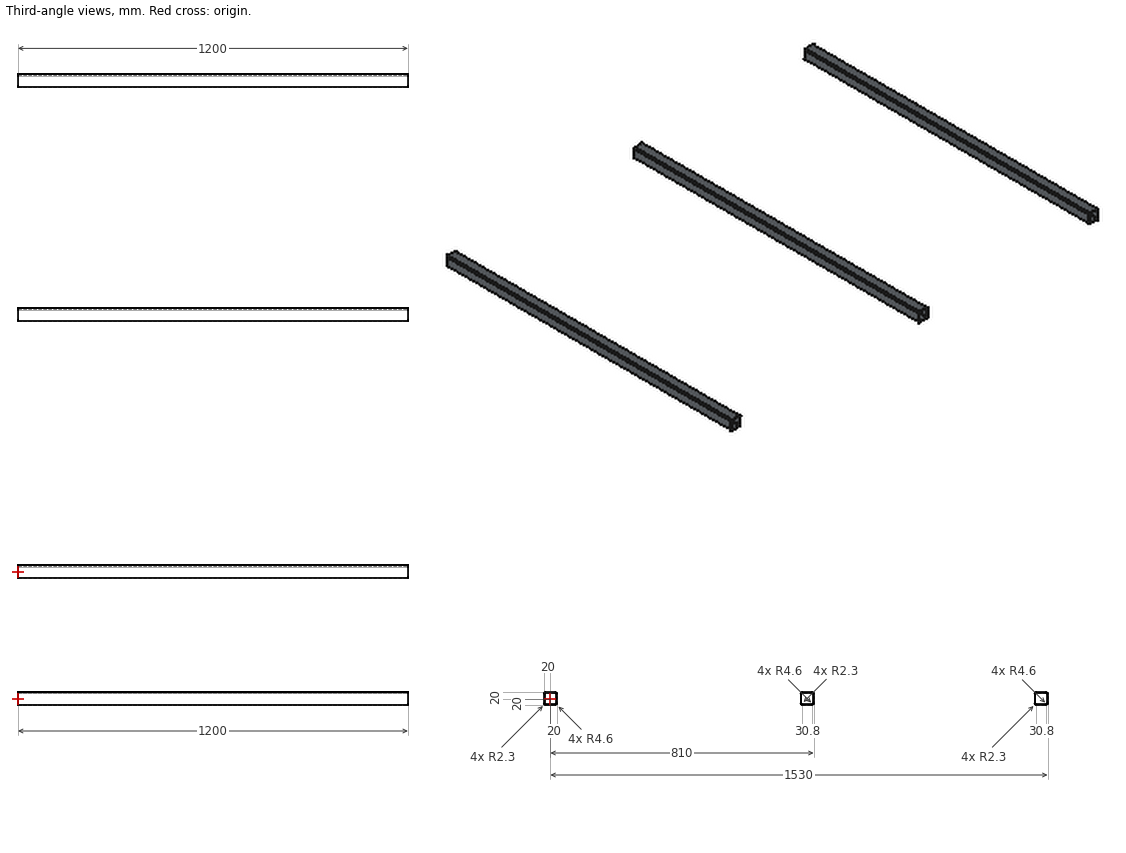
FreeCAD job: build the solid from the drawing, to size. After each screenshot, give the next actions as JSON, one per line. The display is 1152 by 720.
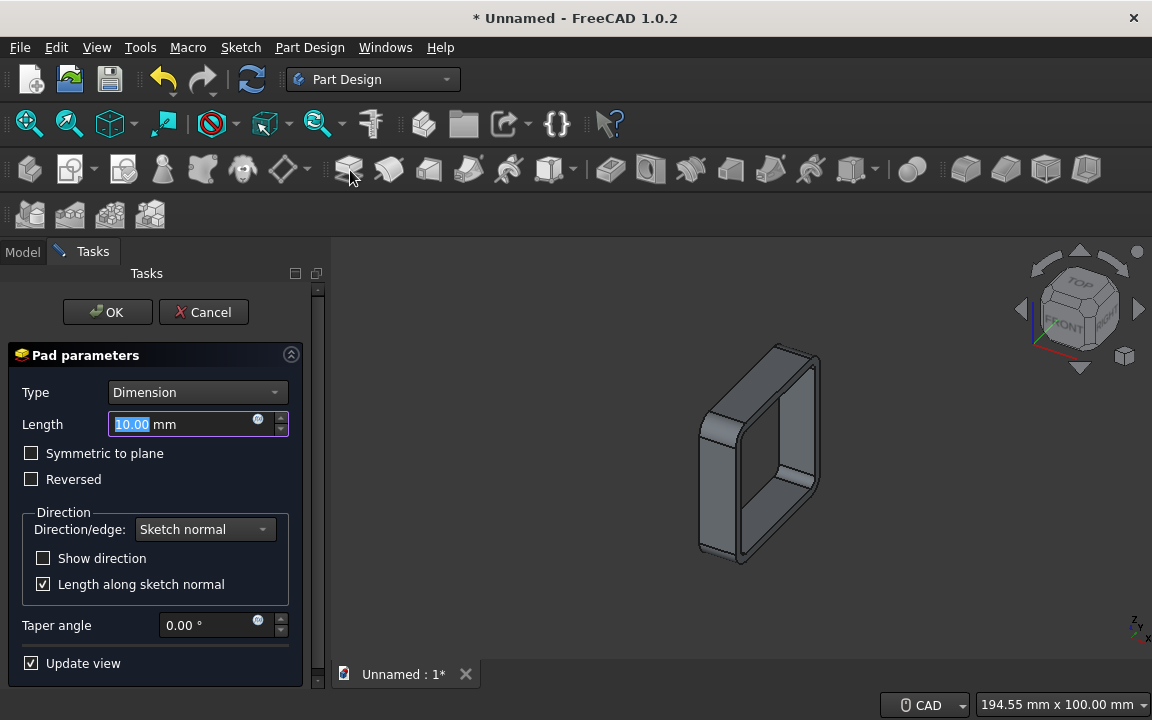
{"action": "type", "text": "1200"}
{"action": "key", "text": "Tab"}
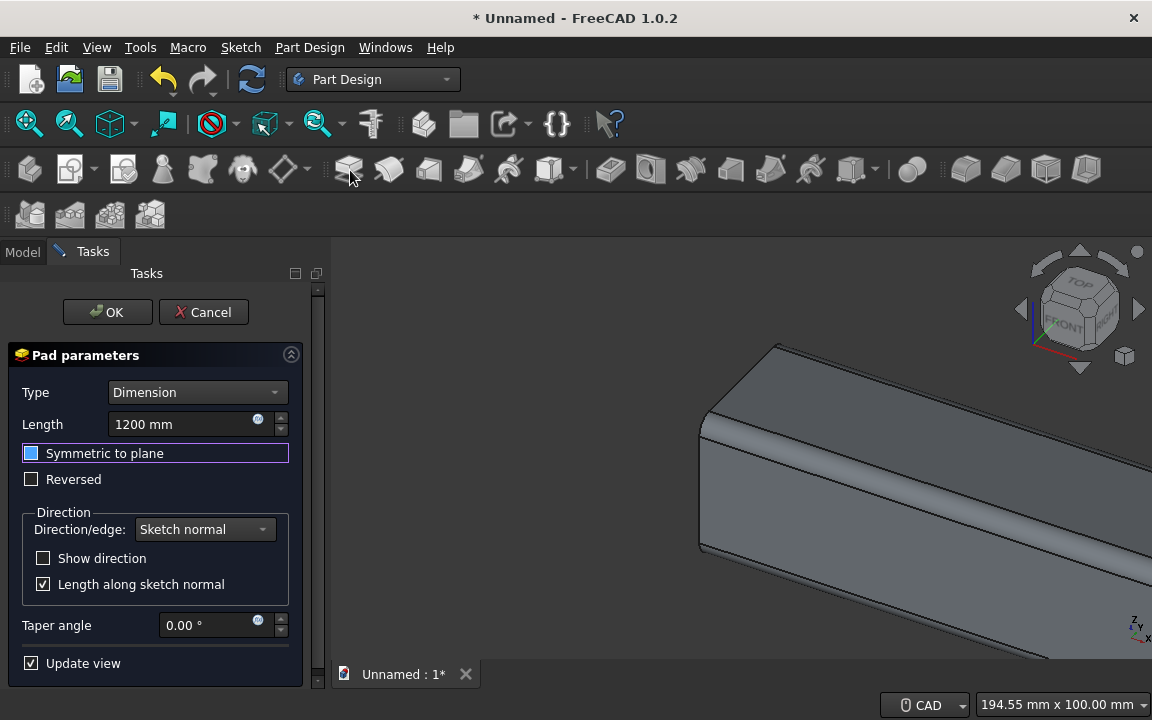
{"action": "left_click", "coordinate": [108, 312]}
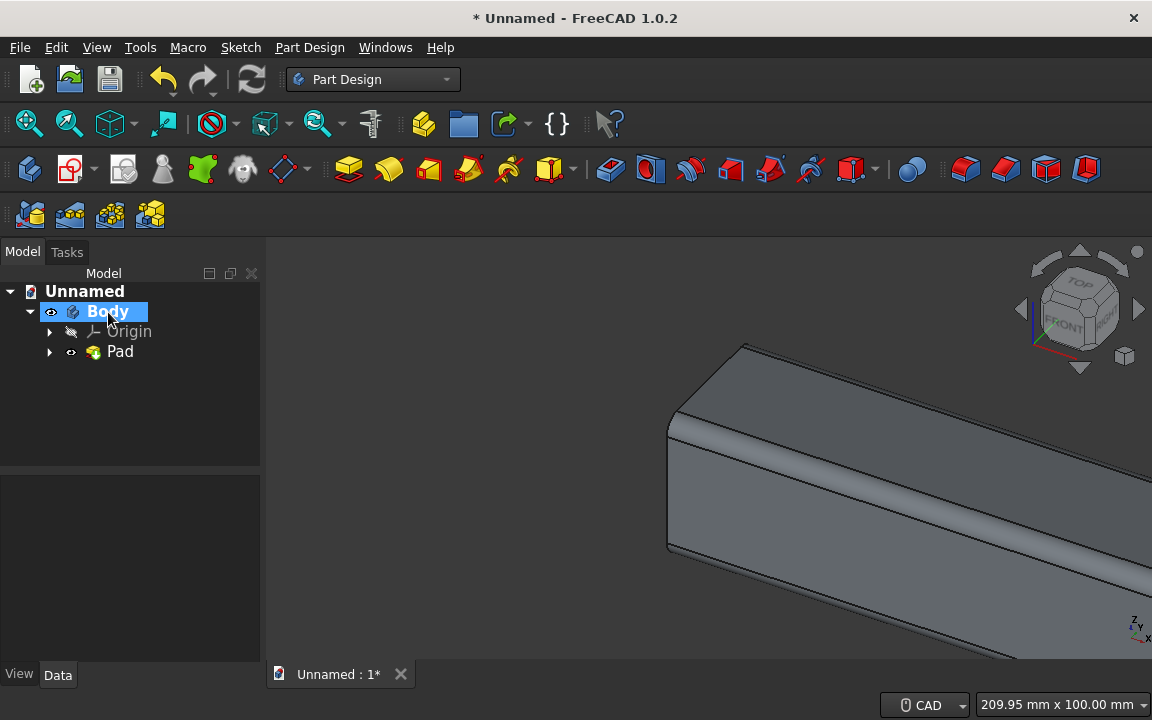
{"action": "key", "text": "v f"}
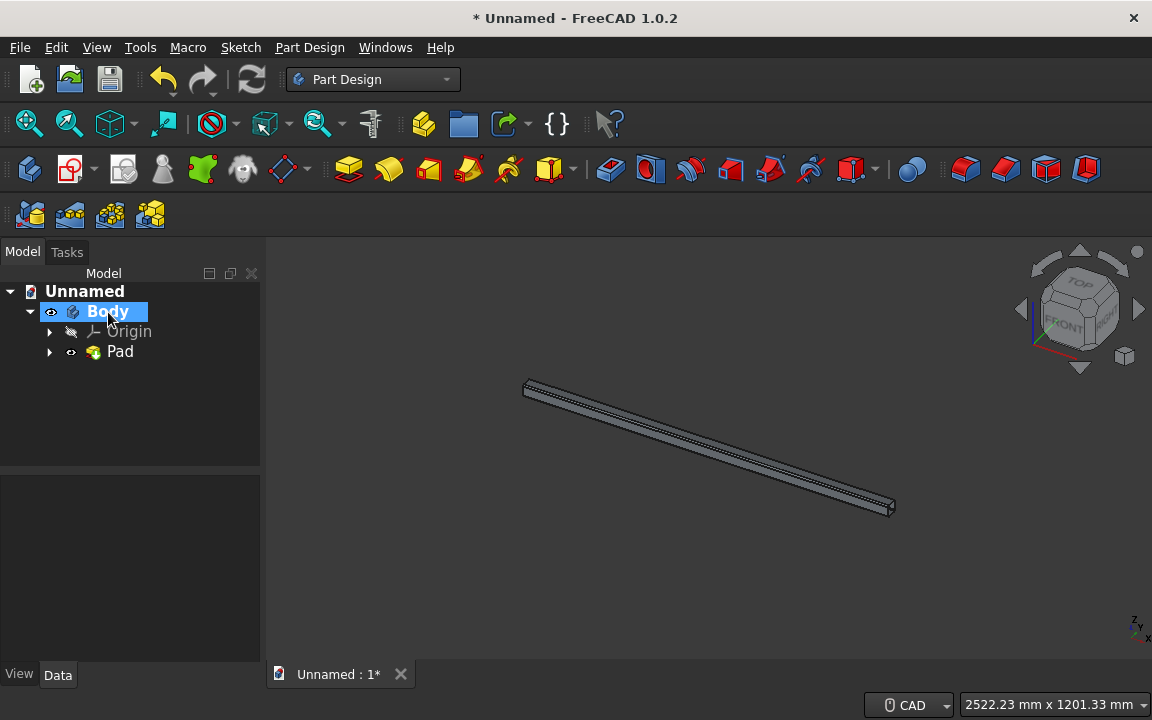
{"action": "left_click", "coordinate": [30, 170]}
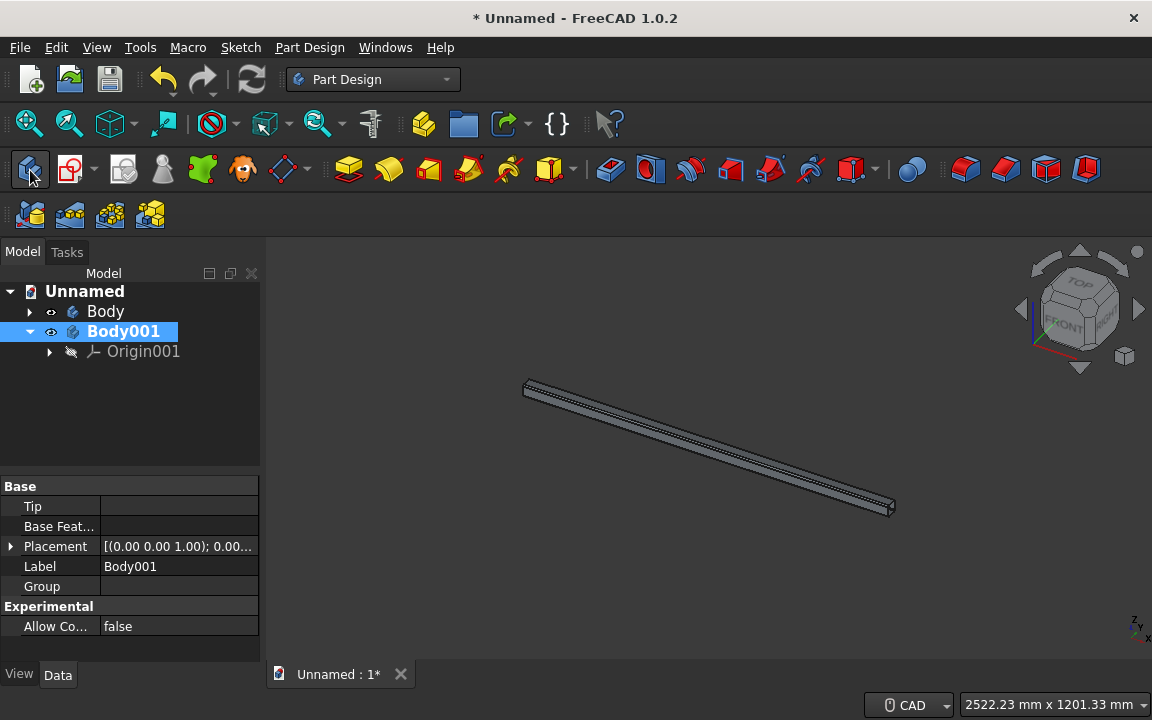
{"action": "left_click", "coordinate": [306, 619]}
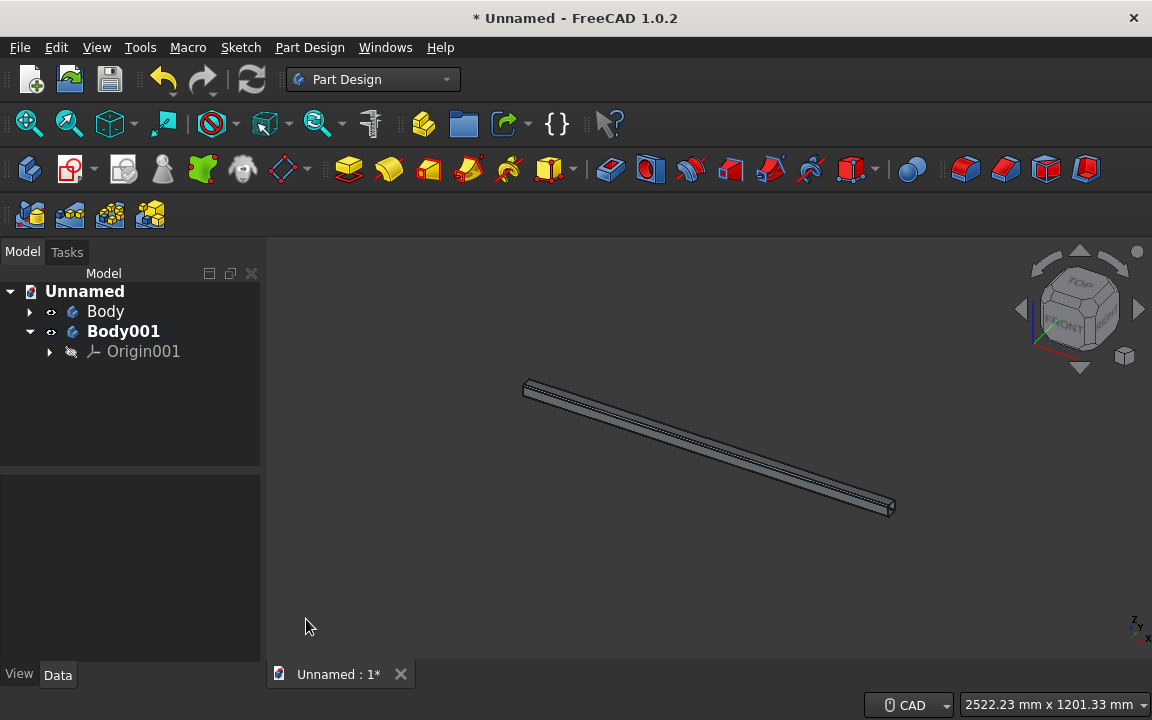
{"action": "left_click", "coordinate": [70, 170]}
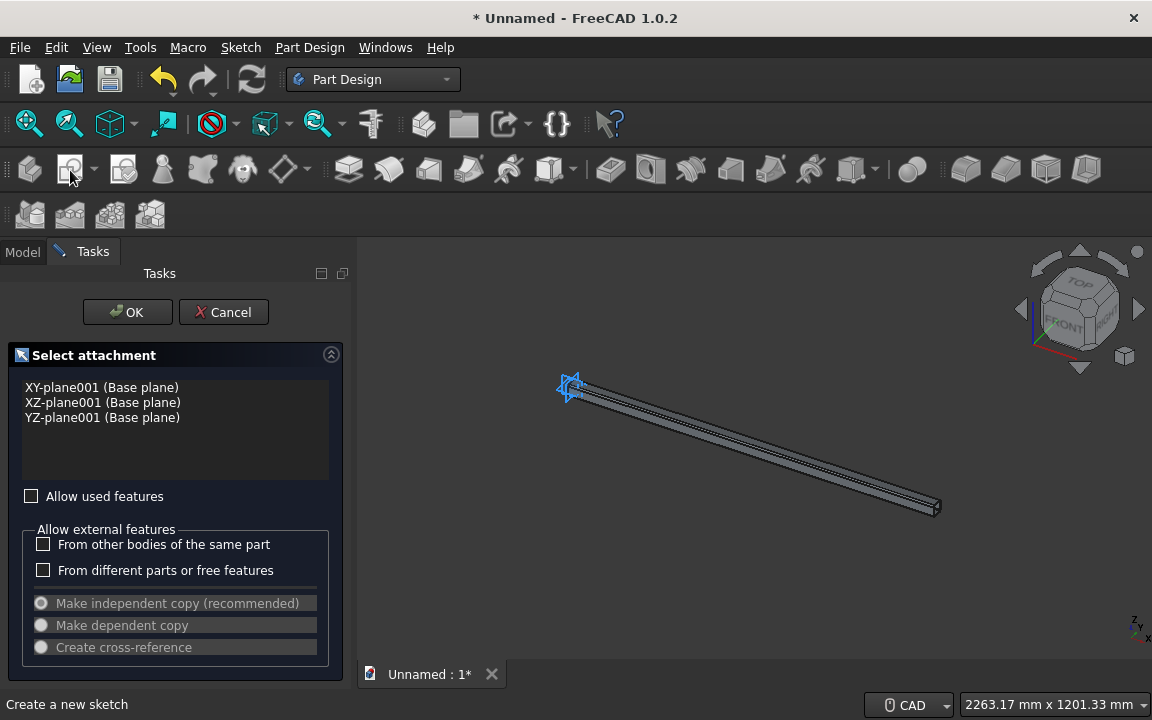
{"action": "left_click", "coordinate": [82, 418]}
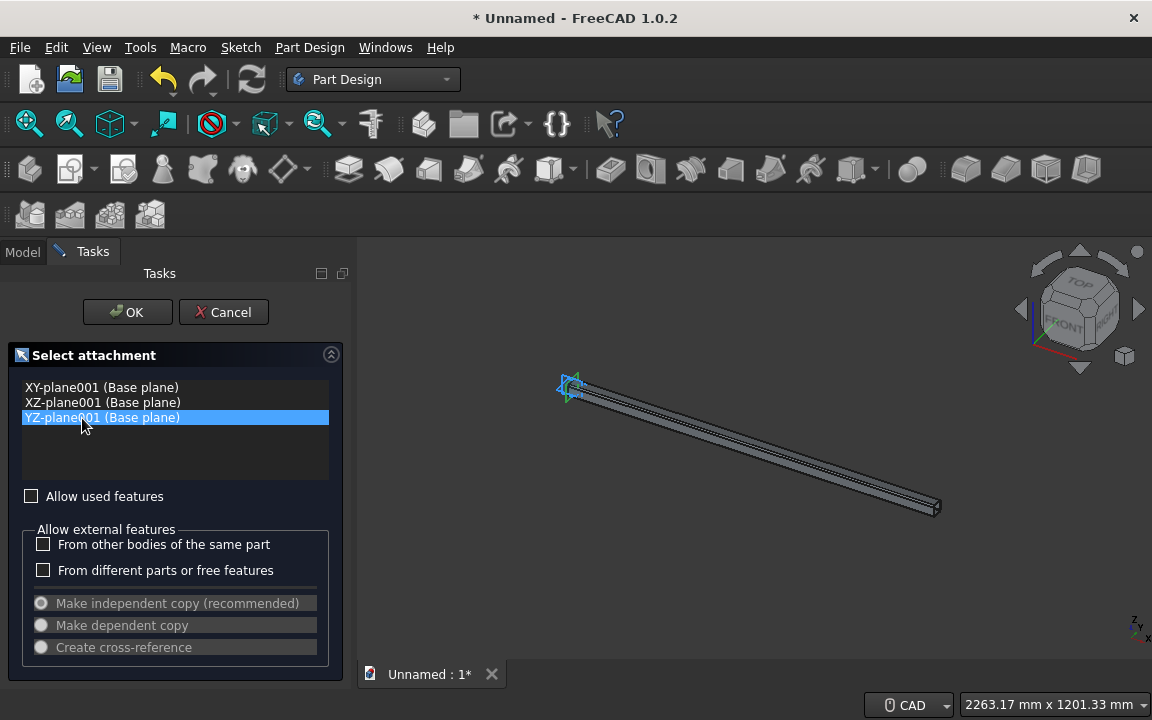
{"action": "left_click", "coordinate": [128, 312]}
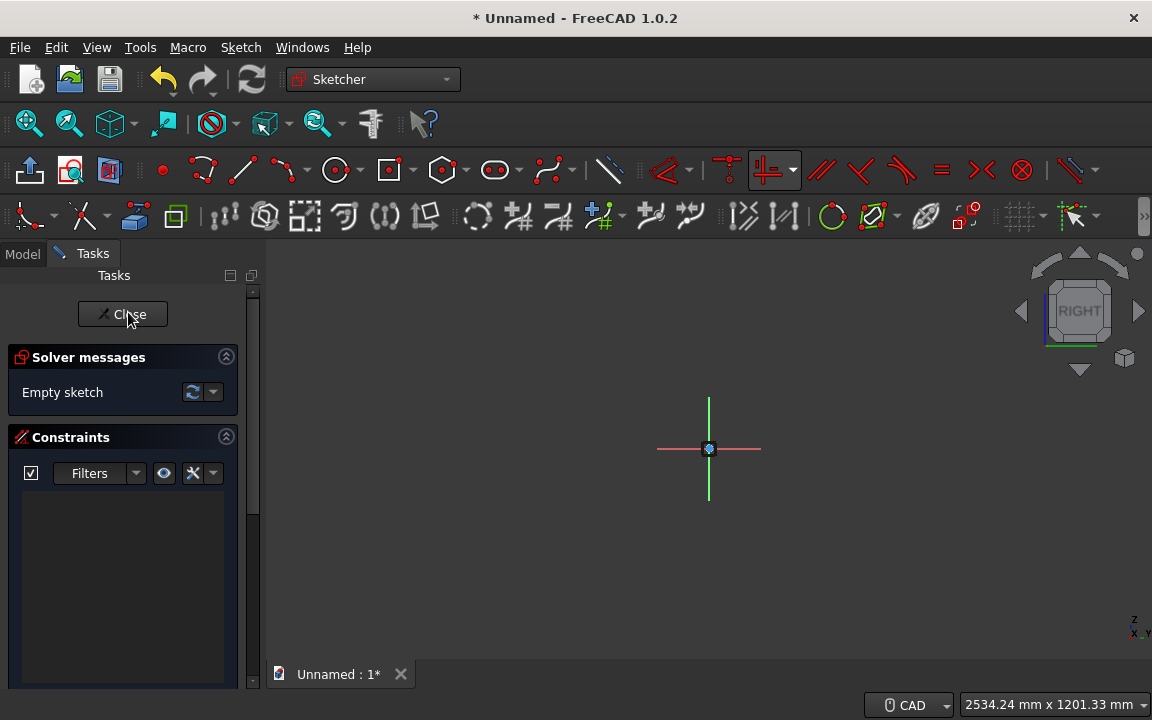
{"action": "scroll", "coordinate": [640, 449], "scroll_direction": "down", "scroll_amount": 5}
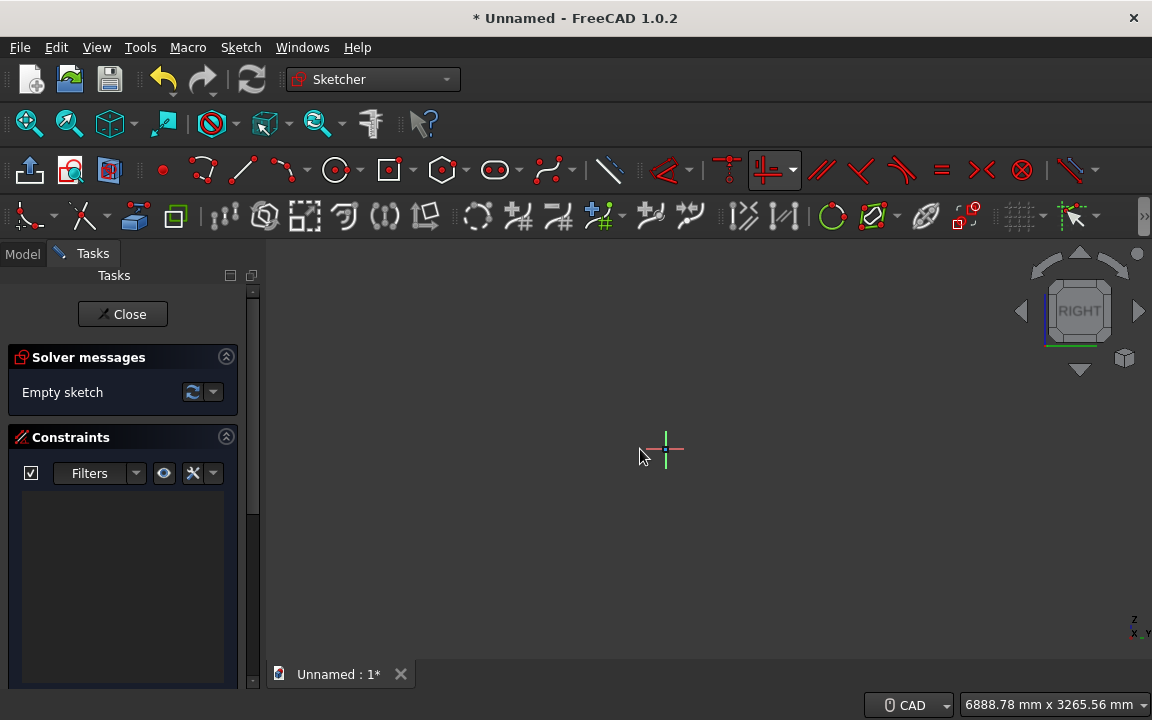
{"action": "scroll", "coordinate": [871, 449], "scroll_direction": "up", "scroll_amount": 15}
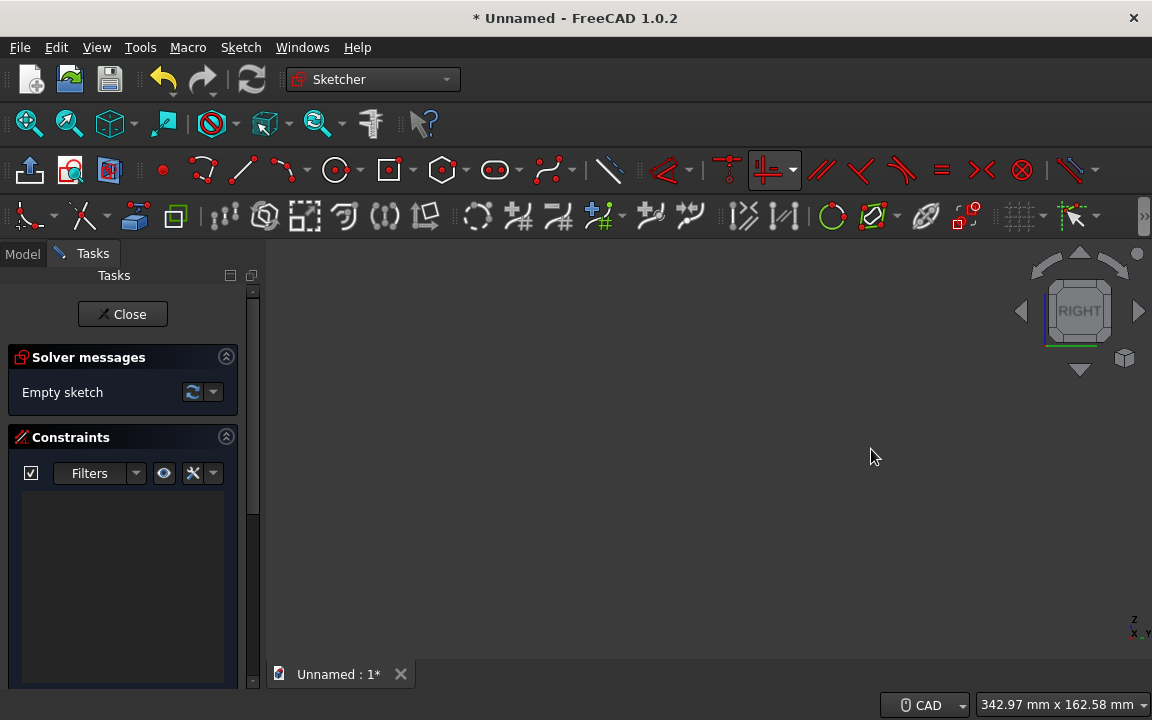
{"action": "scroll", "coordinate": [631, 444], "scroll_direction": "up", "scroll_amount": 5}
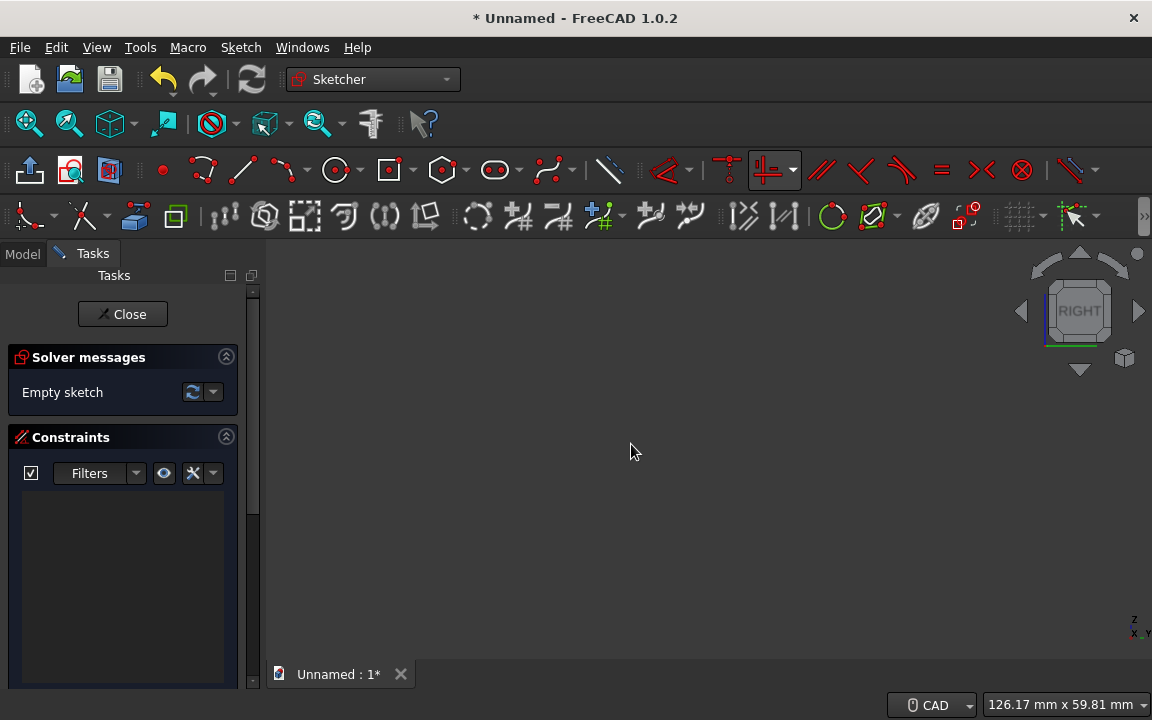
{"action": "left_click", "coordinate": [244, 170]}